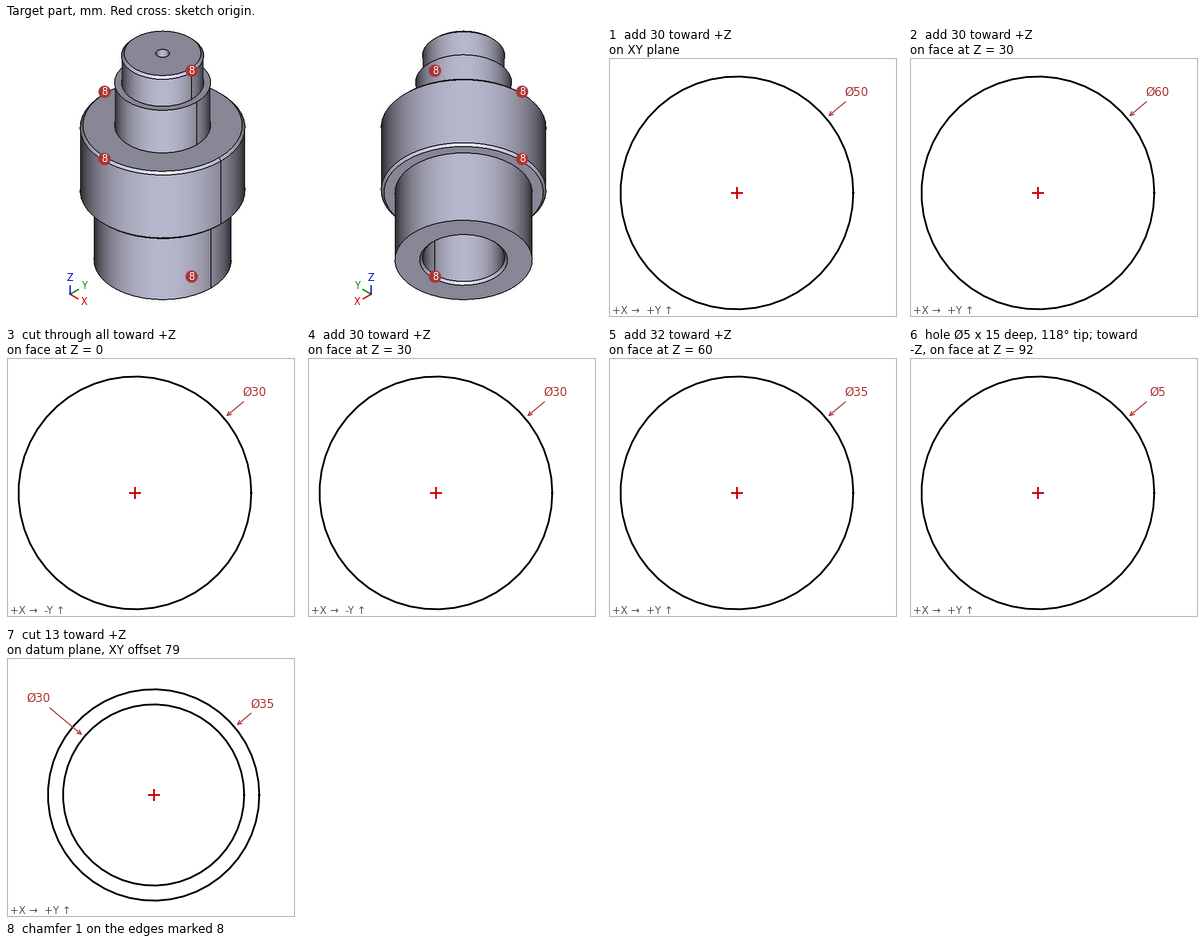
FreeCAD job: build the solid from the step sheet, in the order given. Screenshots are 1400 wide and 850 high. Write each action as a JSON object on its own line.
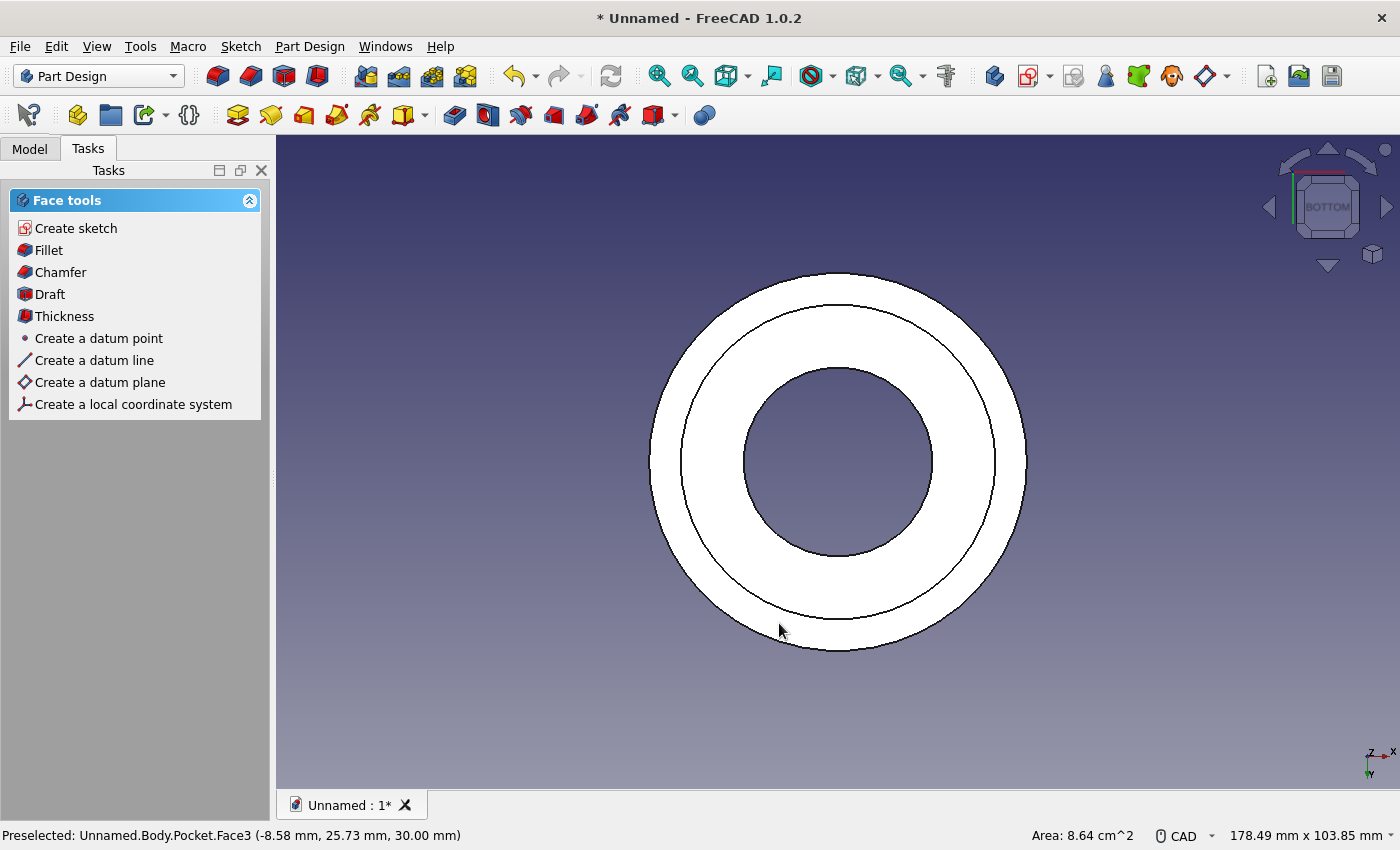
{"action": "left_click", "coordinate": [1028, 76]}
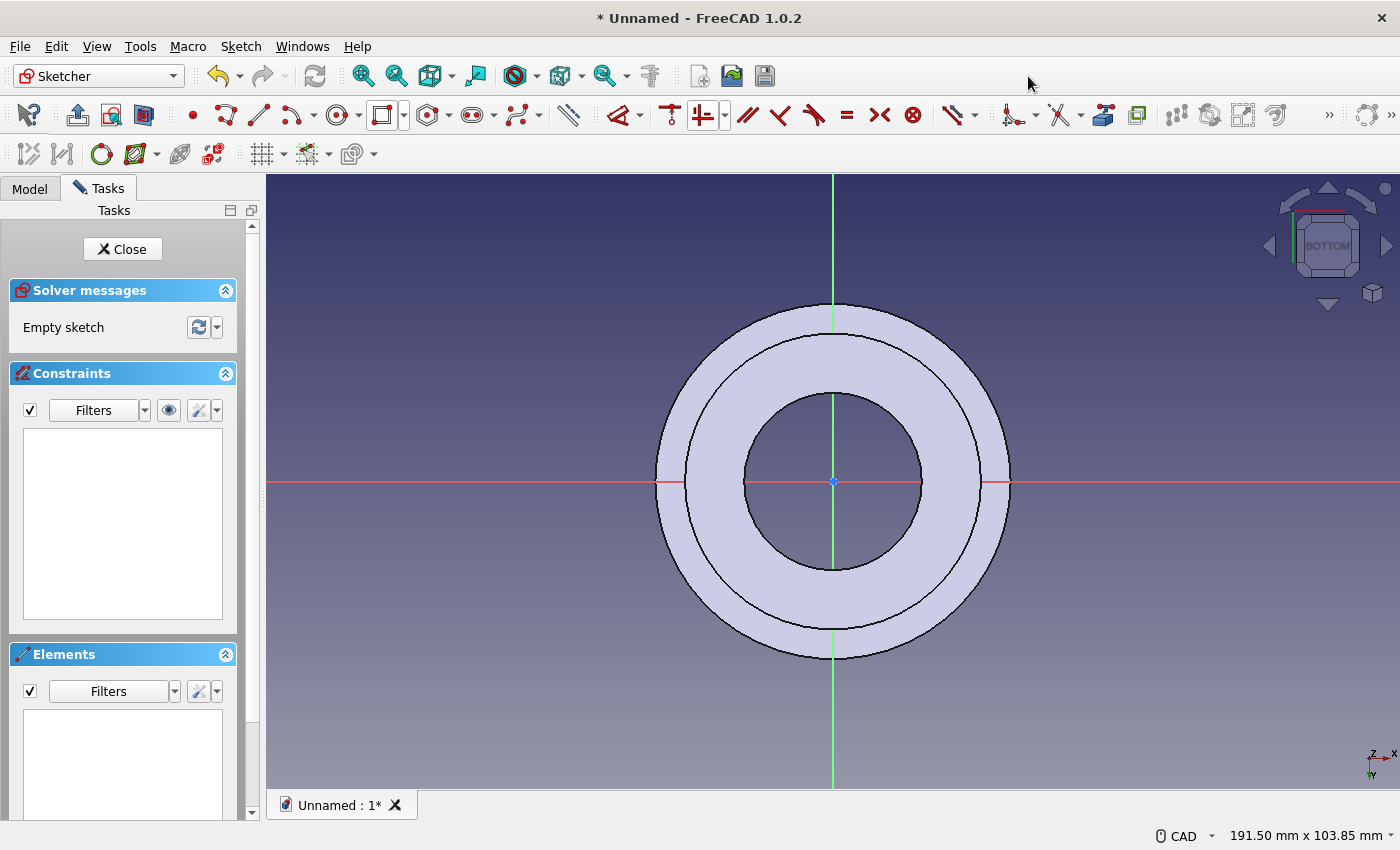
{"action": "scroll", "coordinate": [889, 482], "scroll_direction": "up", "scroll_amount": 4}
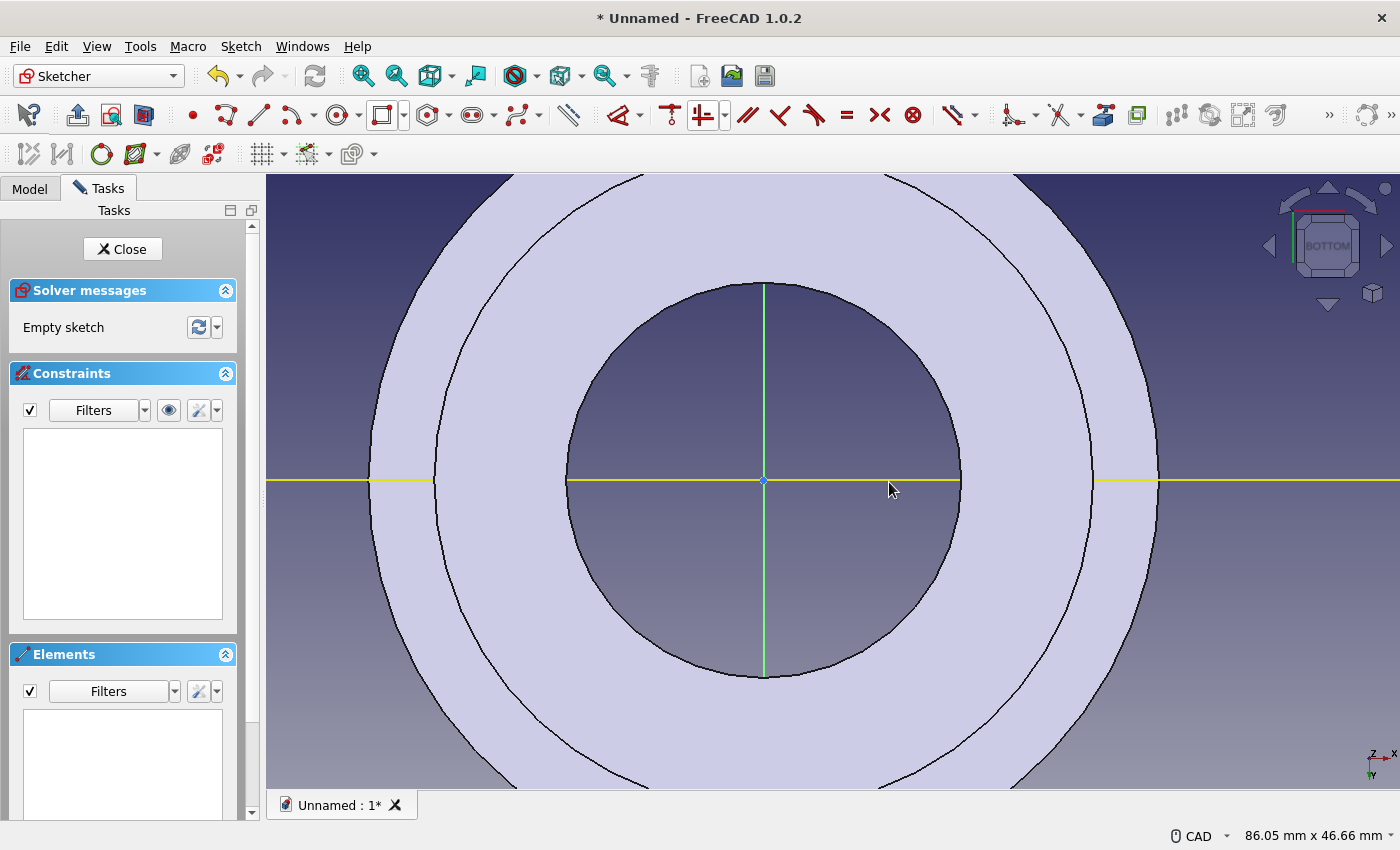
{"action": "key", "text": "g c"}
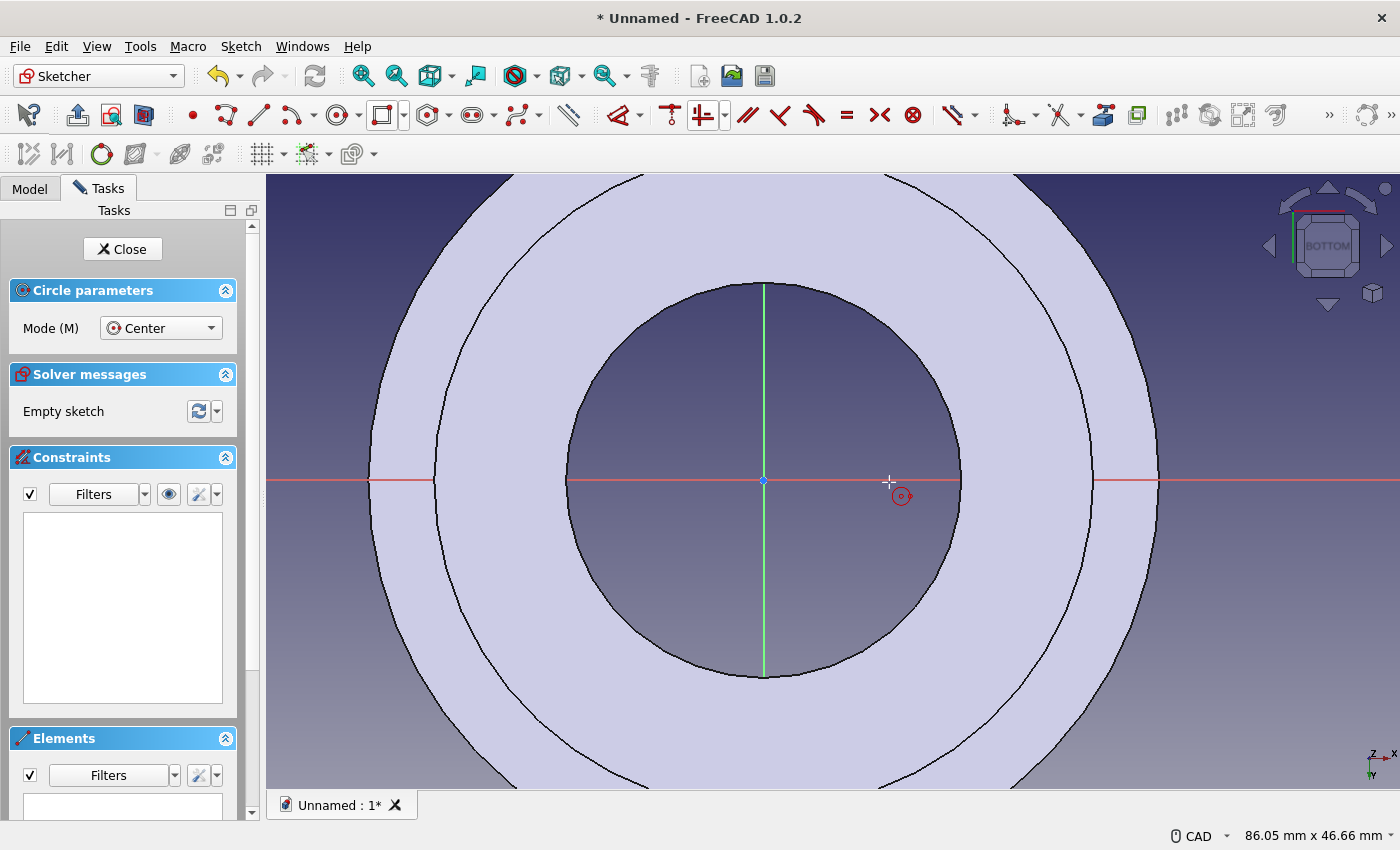
{"action": "left_click", "coordinate": [764, 480]}
{"action": "left_click", "coordinate": [903, 340]}
{"action": "key", "text": "Escape"}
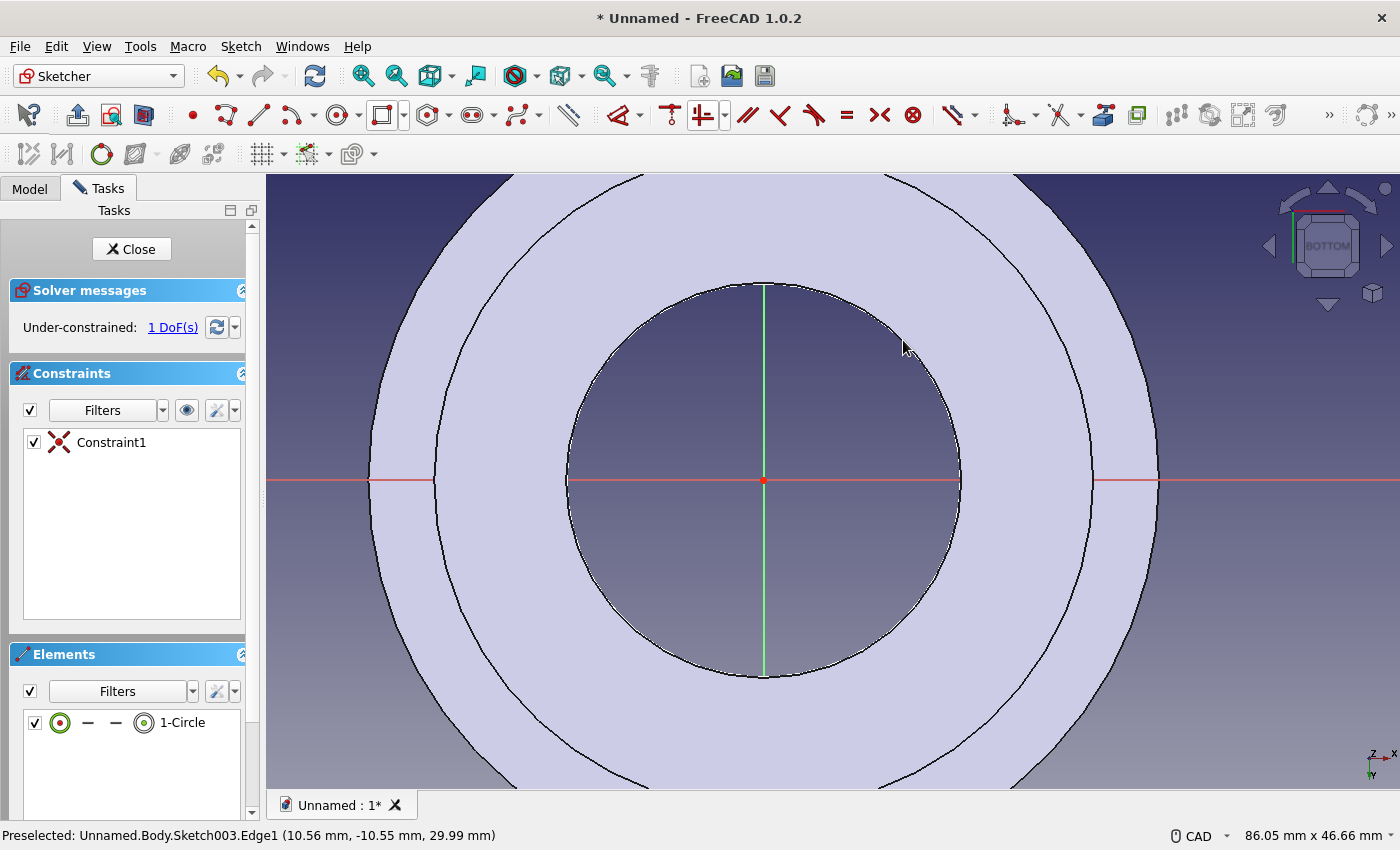
{"action": "key", "text": "d"}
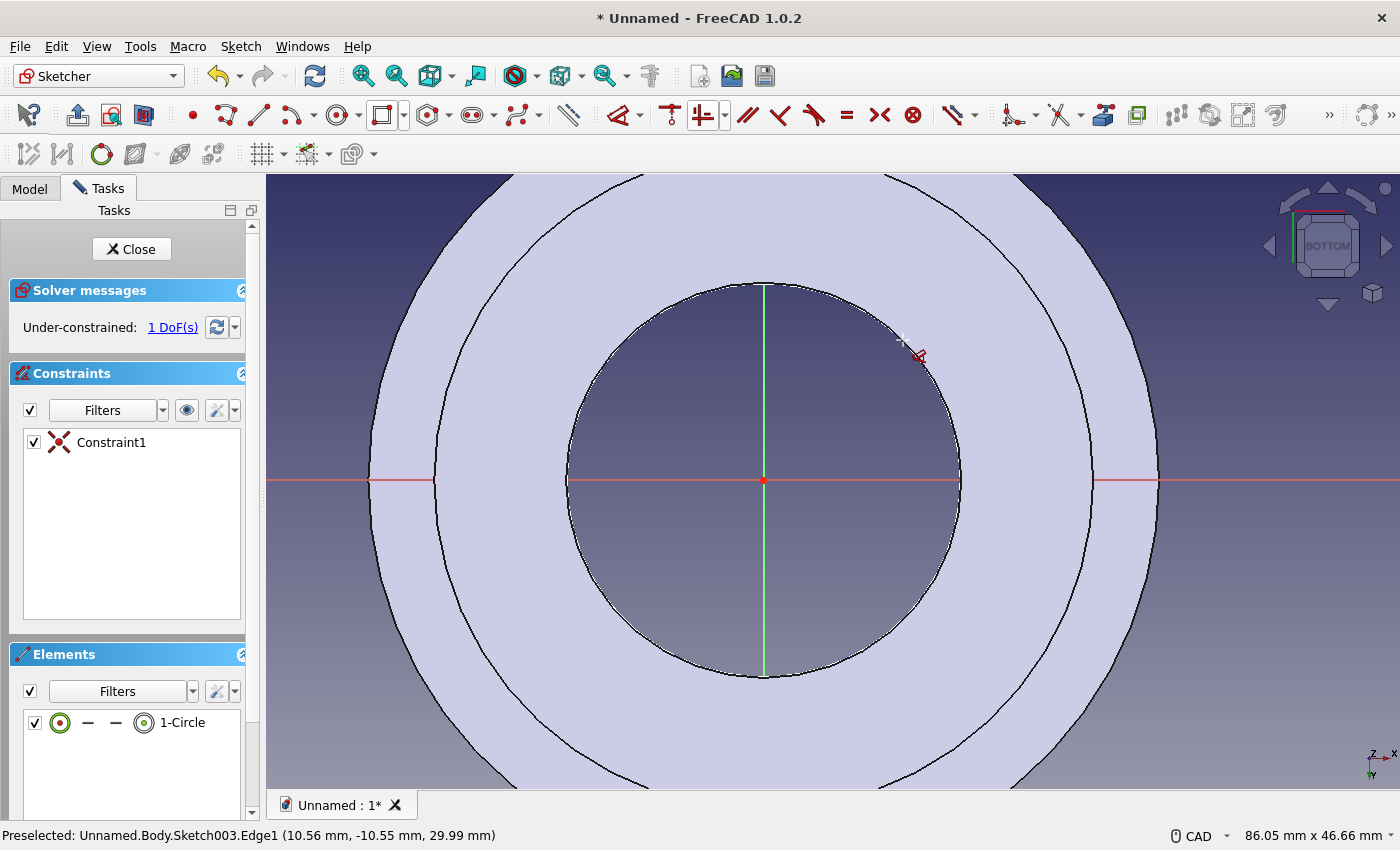
{"action": "left_click", "coordinate": [903, 341]}
{"action": "left_click", "coordinate": [926, 318]}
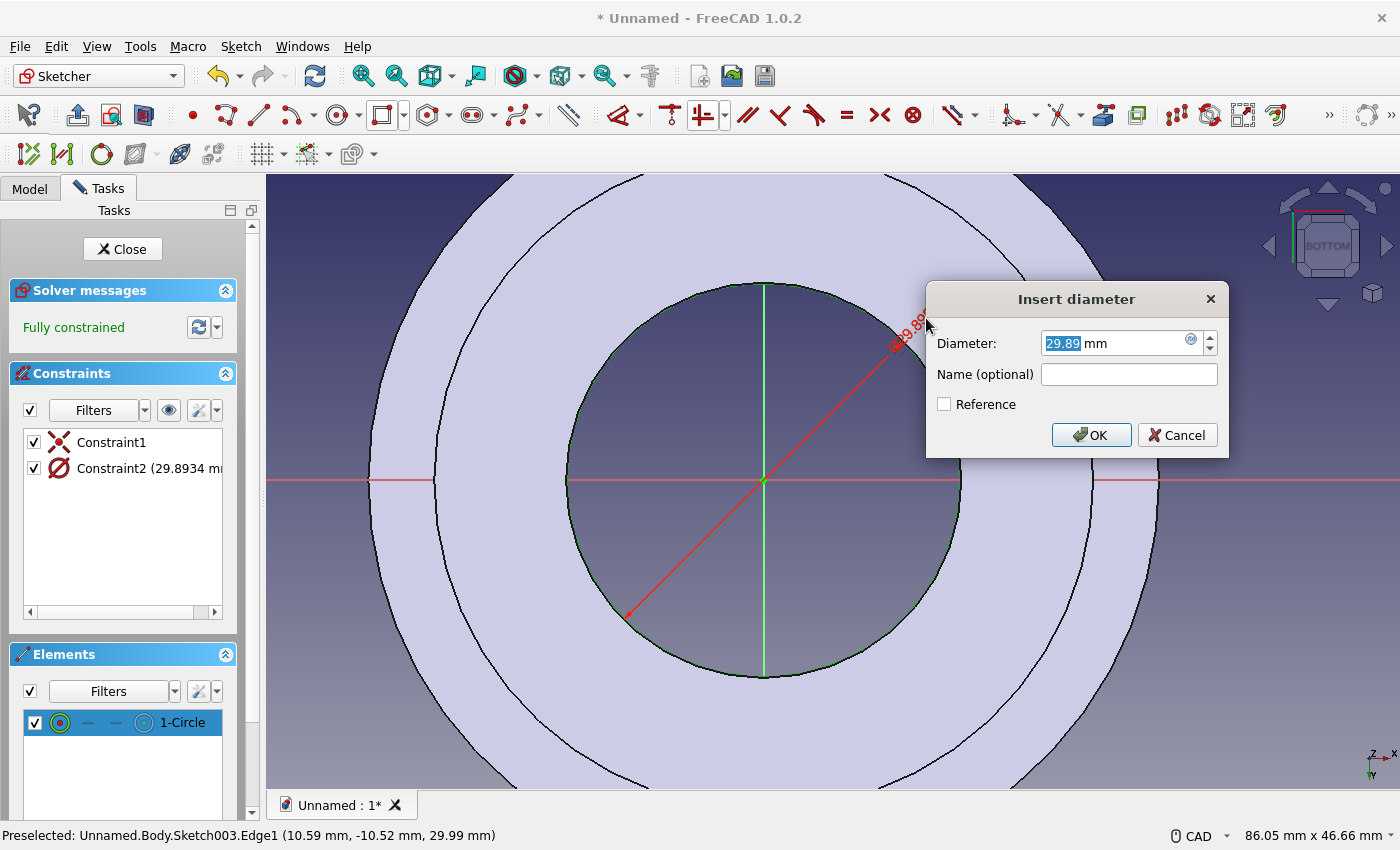
{"action": "type", "text": "30"}
{"action": "key", "text": "Return"}
{"action": "key", "text": "Escape"}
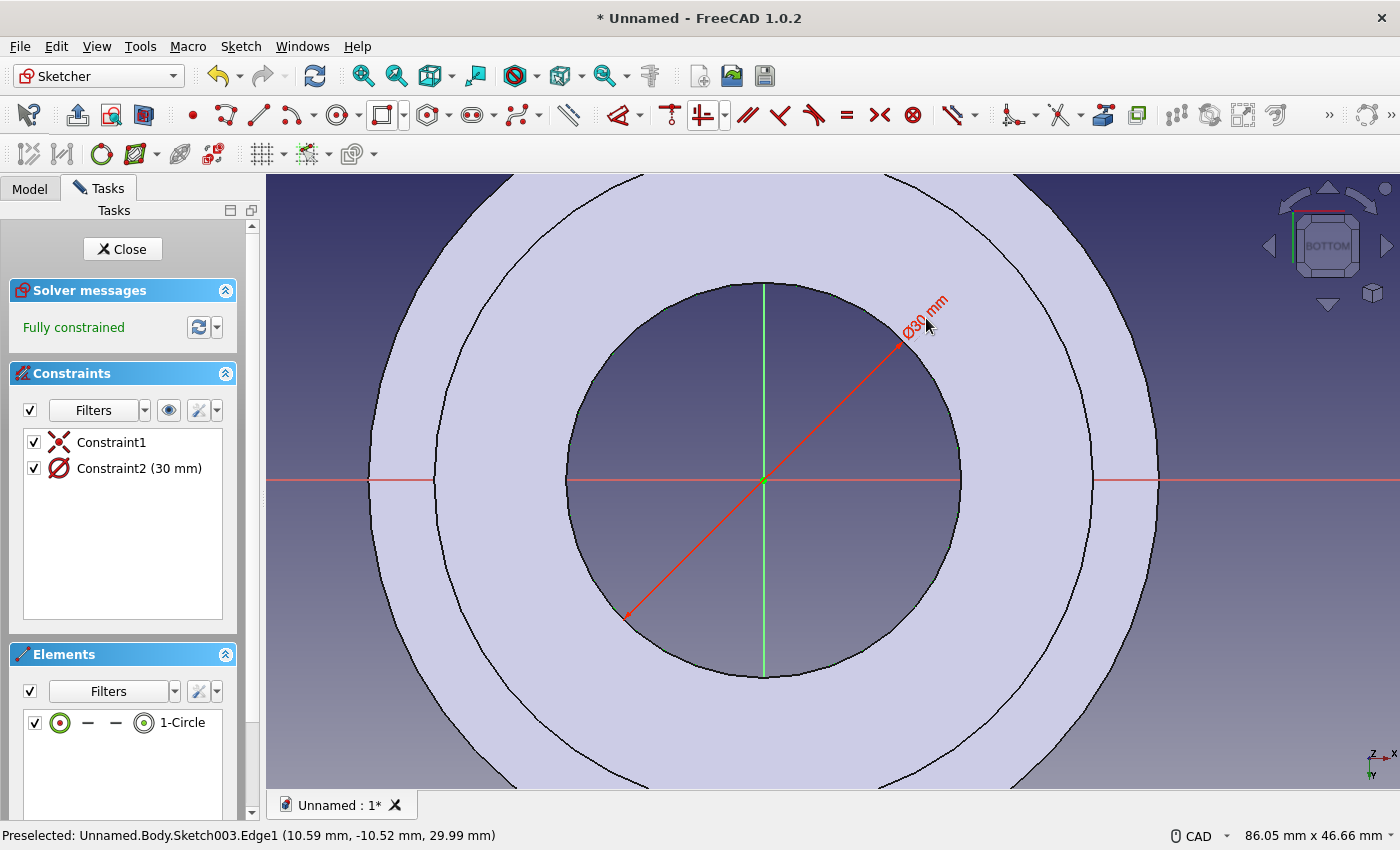
{"action": "left_click", "coordinate": [123, 249]}